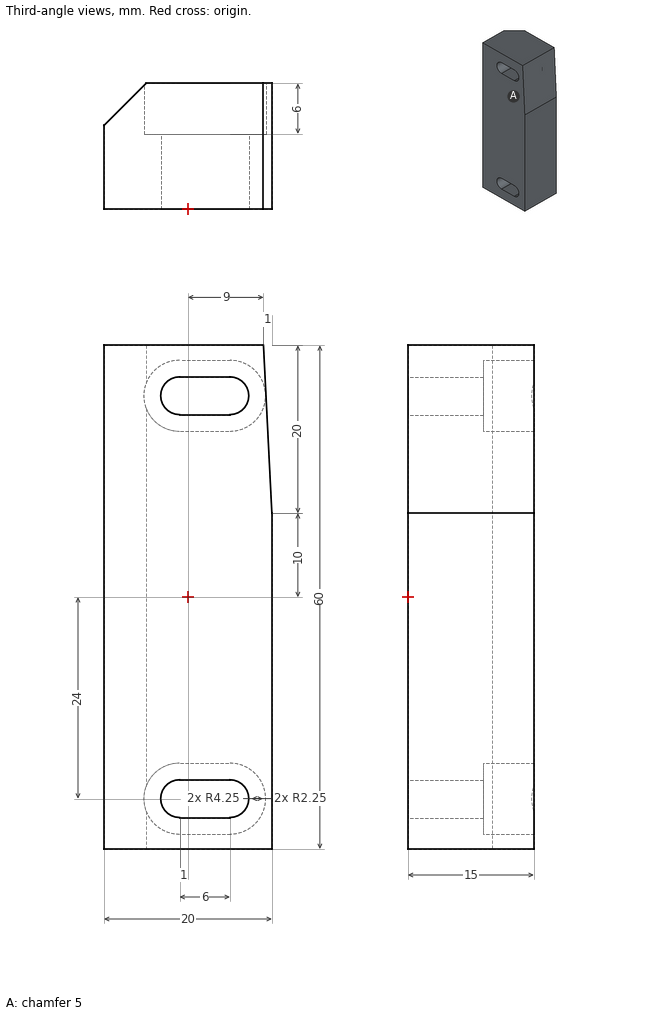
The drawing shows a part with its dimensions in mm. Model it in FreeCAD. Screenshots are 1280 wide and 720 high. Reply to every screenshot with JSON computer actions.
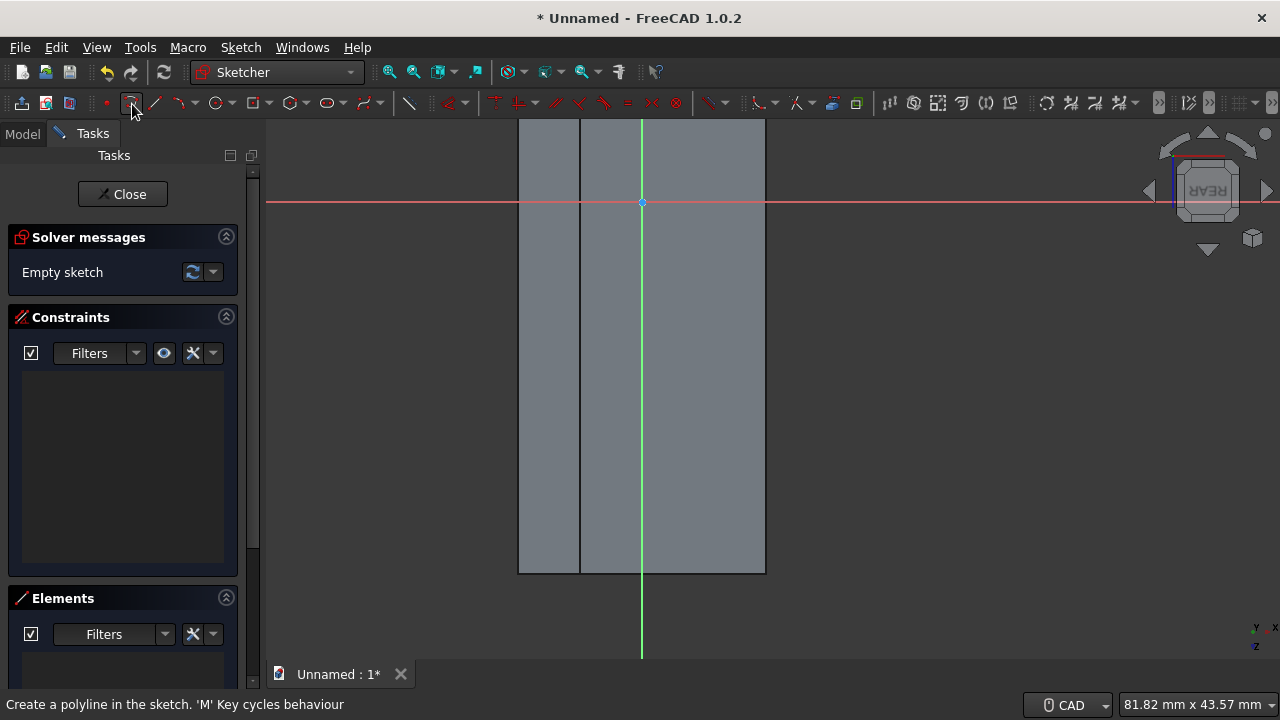
{"action": "left_click", "coordinate": [766, 326]}
{"action": "left_click", "coordinate": [753, 574]}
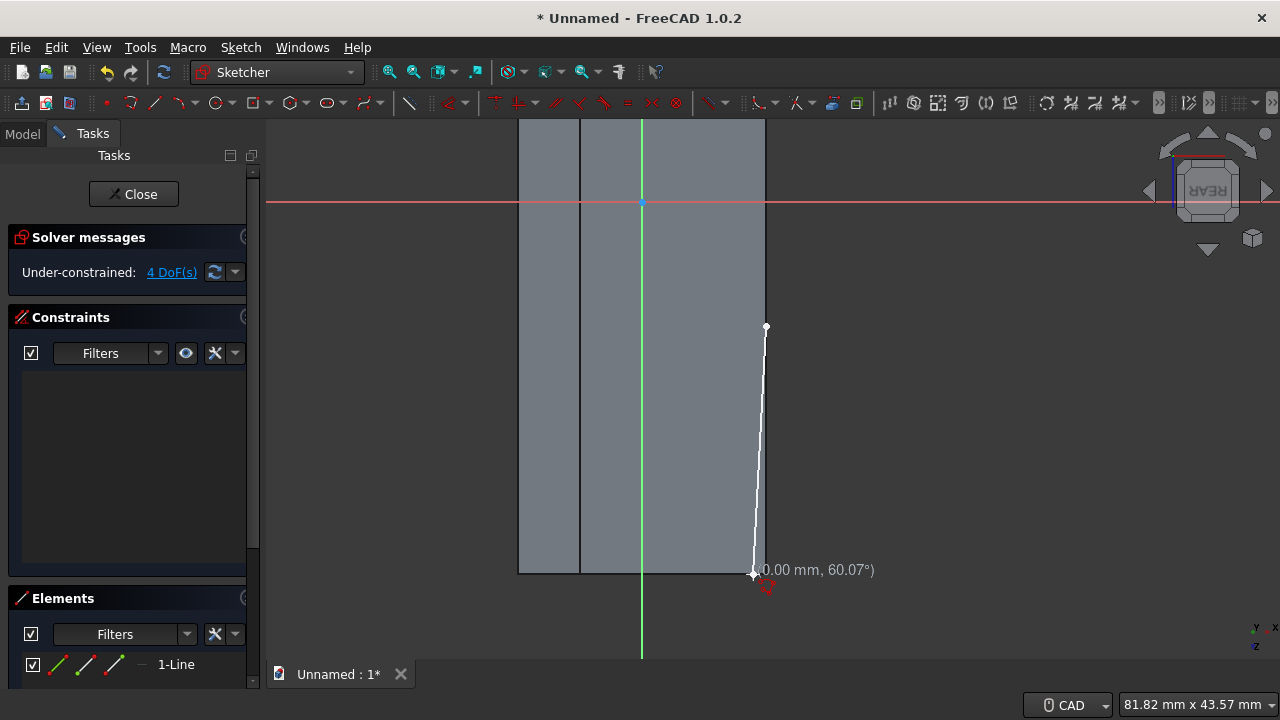
{"action": "scroll", "coordinate": [766, 574], "scroll_direction": "up", "scroll_amount": 2}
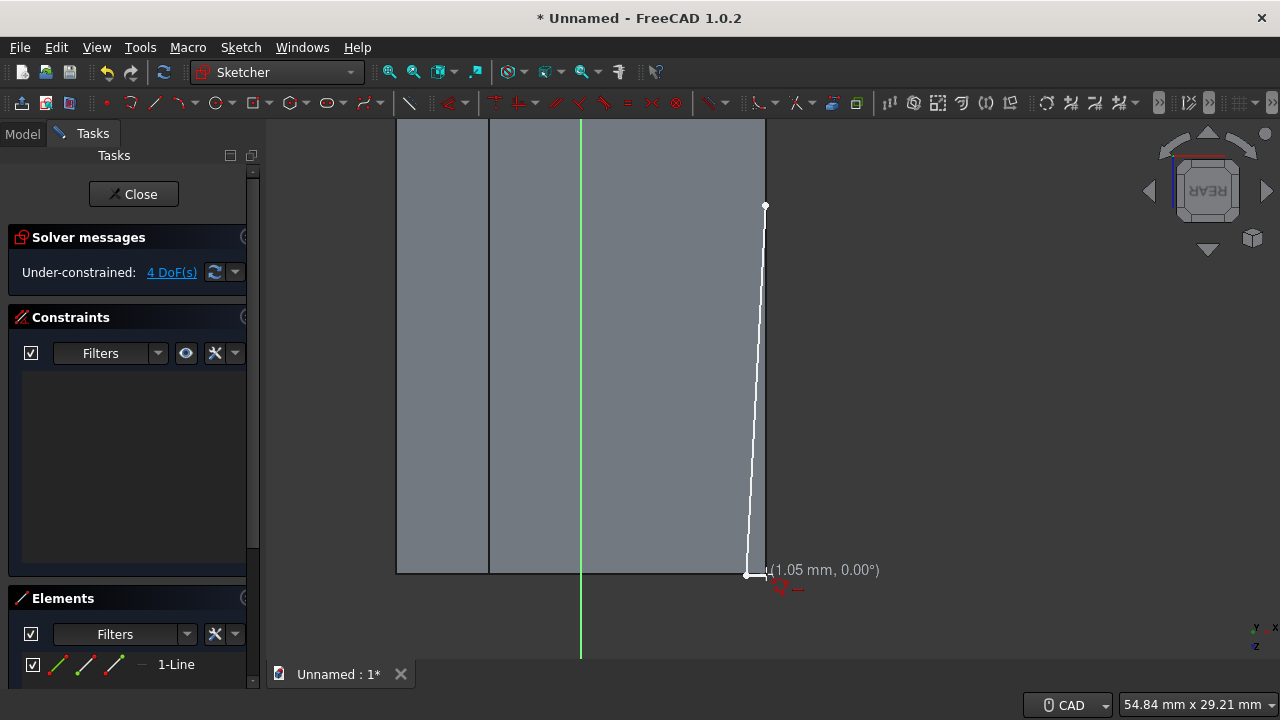
{"action": "left_click", "coordinate": [766, 574]}
{"action": "left_click", "coordinate": [766, 205]}
{"action": "key", "text": "Escape"}
{"action": "key", "text": "Escape"}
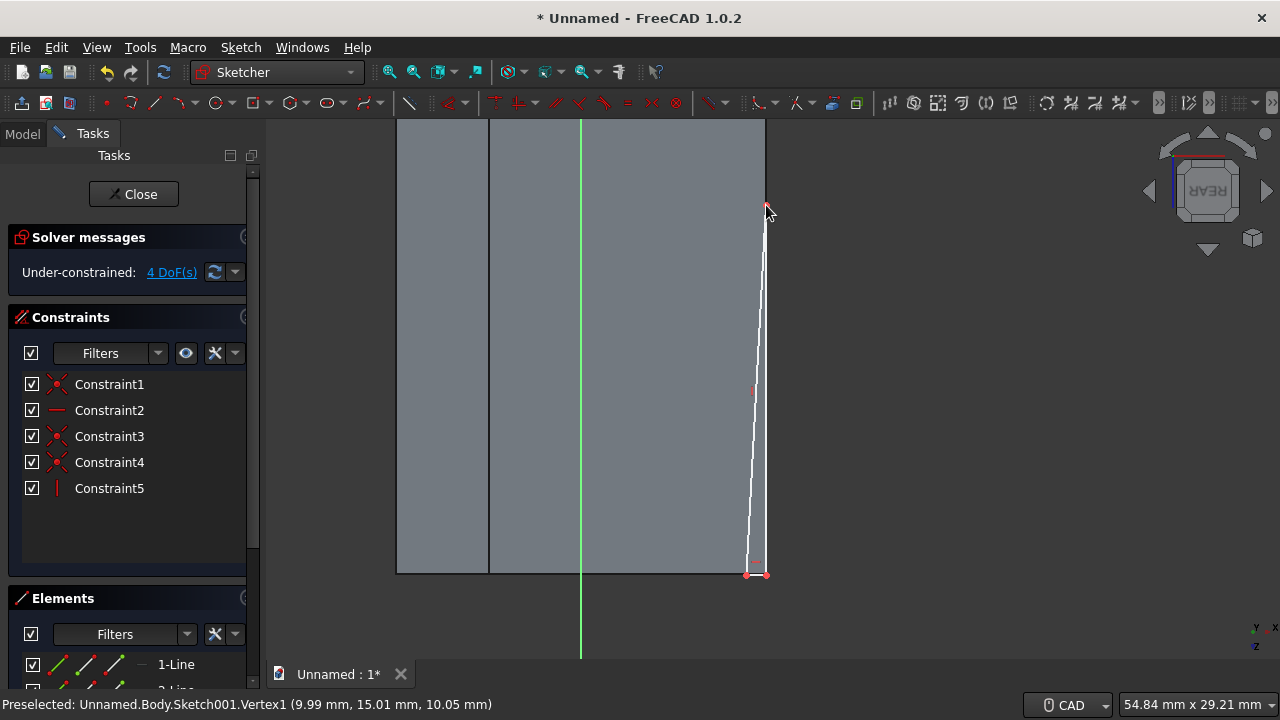
{"action": "left_click", "coordinate": [448, 104]}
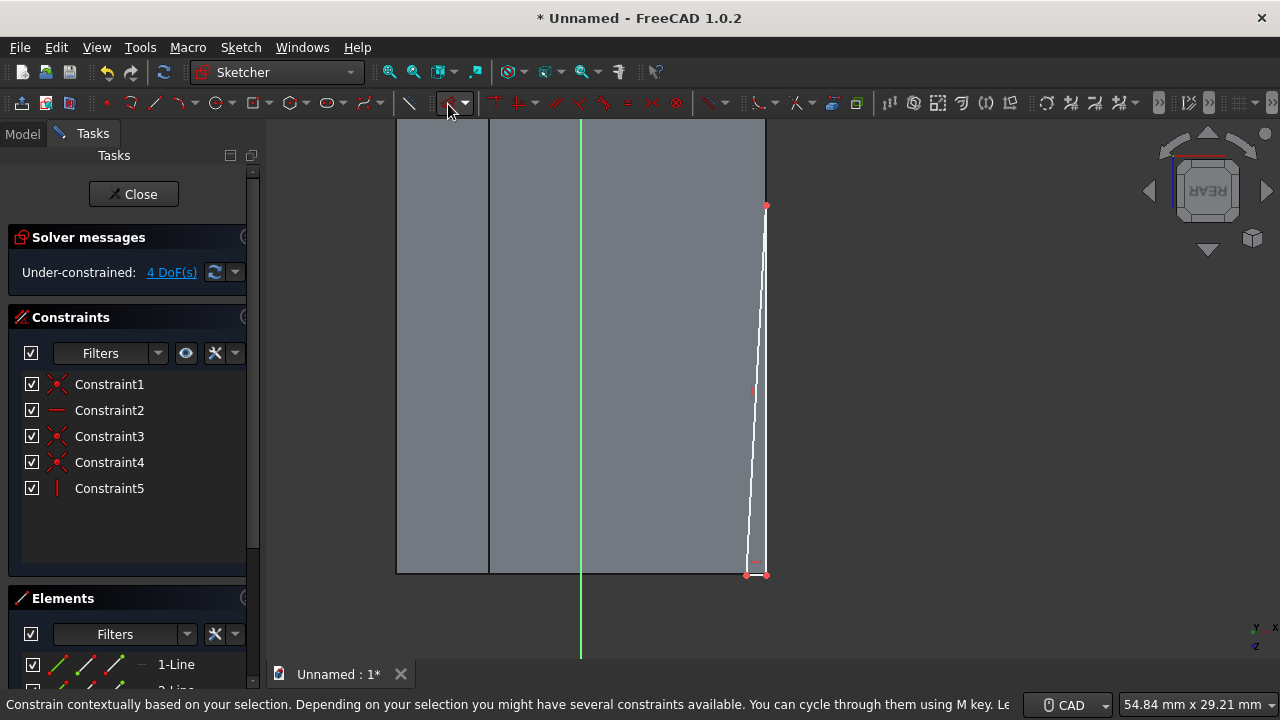
{"action": "scroll", "coordinate": [756, 575], "scroll_direction": "up", "scroll_amount": 4}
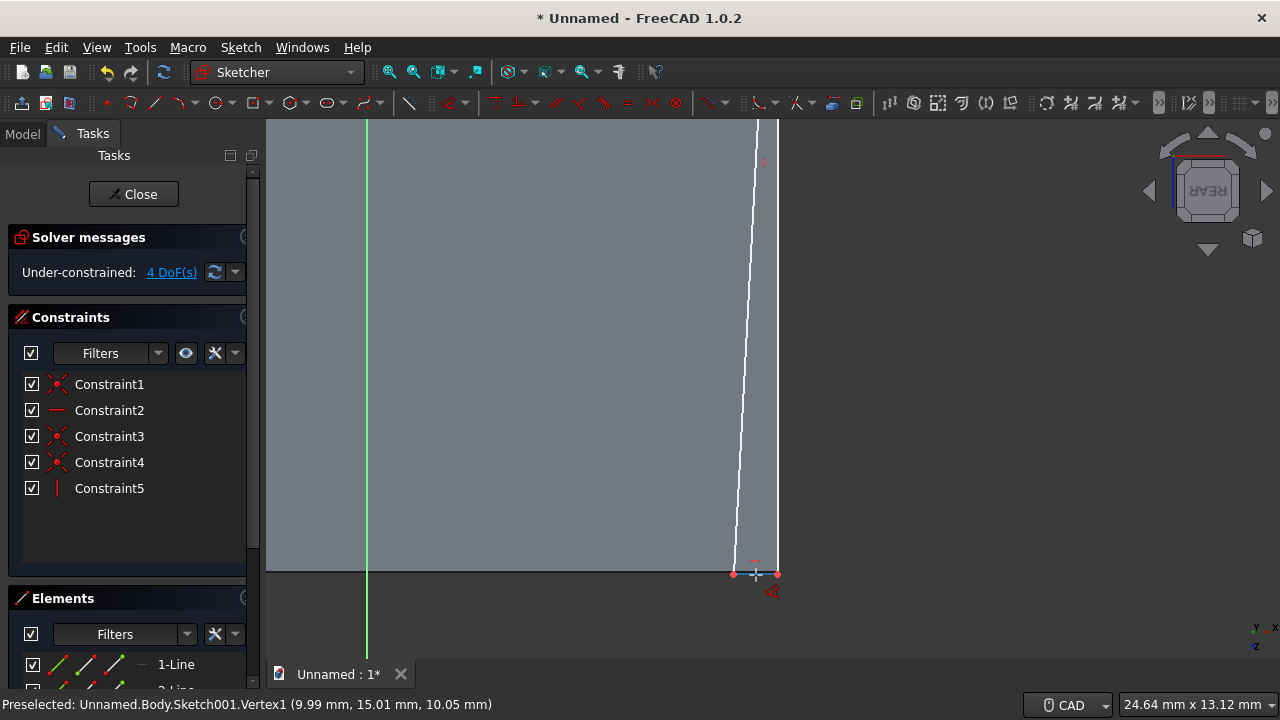
{"action": "left_click", "coordinate": [756, 574]}
{"action": "left_click", "coordinate": [756, 608]}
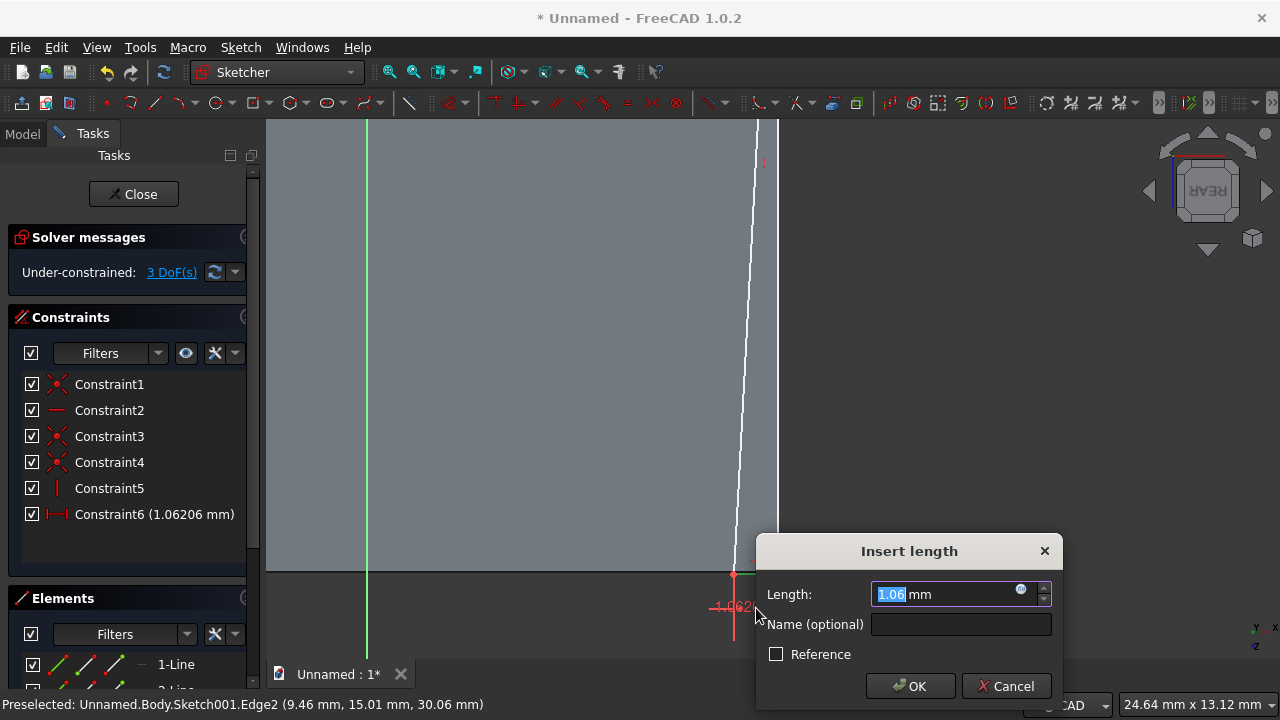
{"action": "type", "text": "1"}
{"action": "key", "text": "Return"}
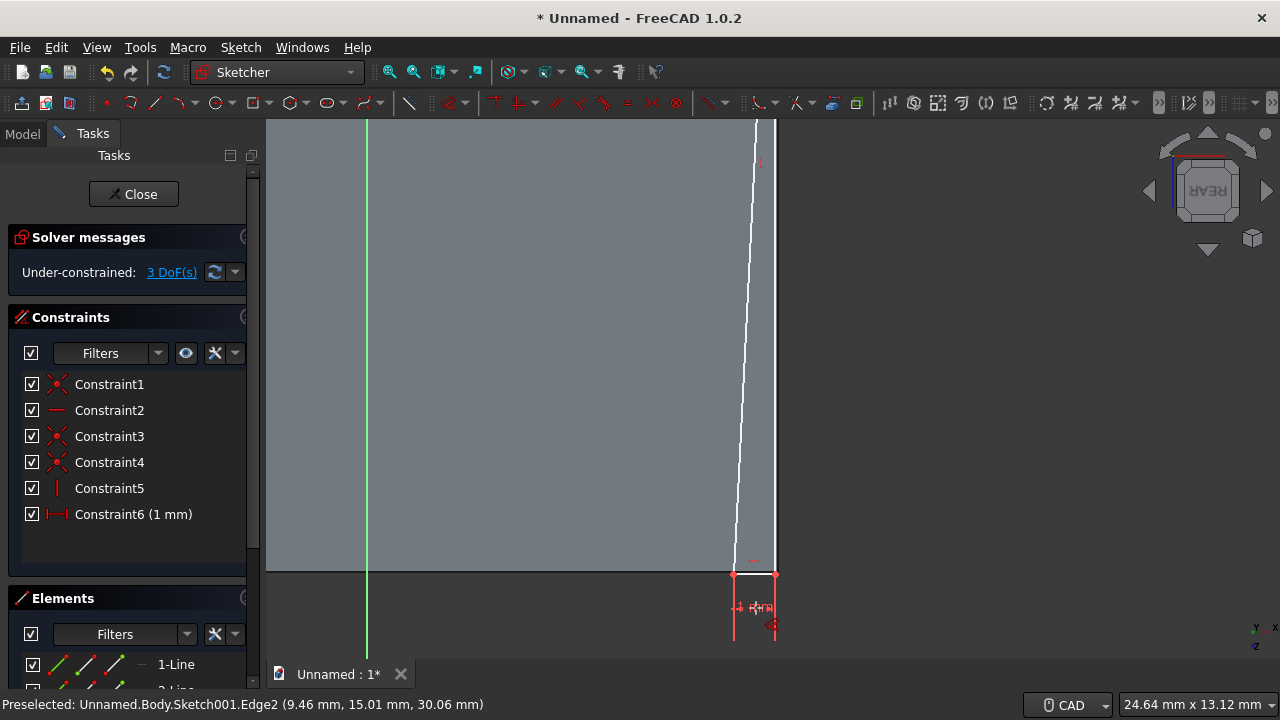
{"action": "left_click", "coordinate": [775, 327]}
{"action": "left_click", "coordinate": [809, 361]}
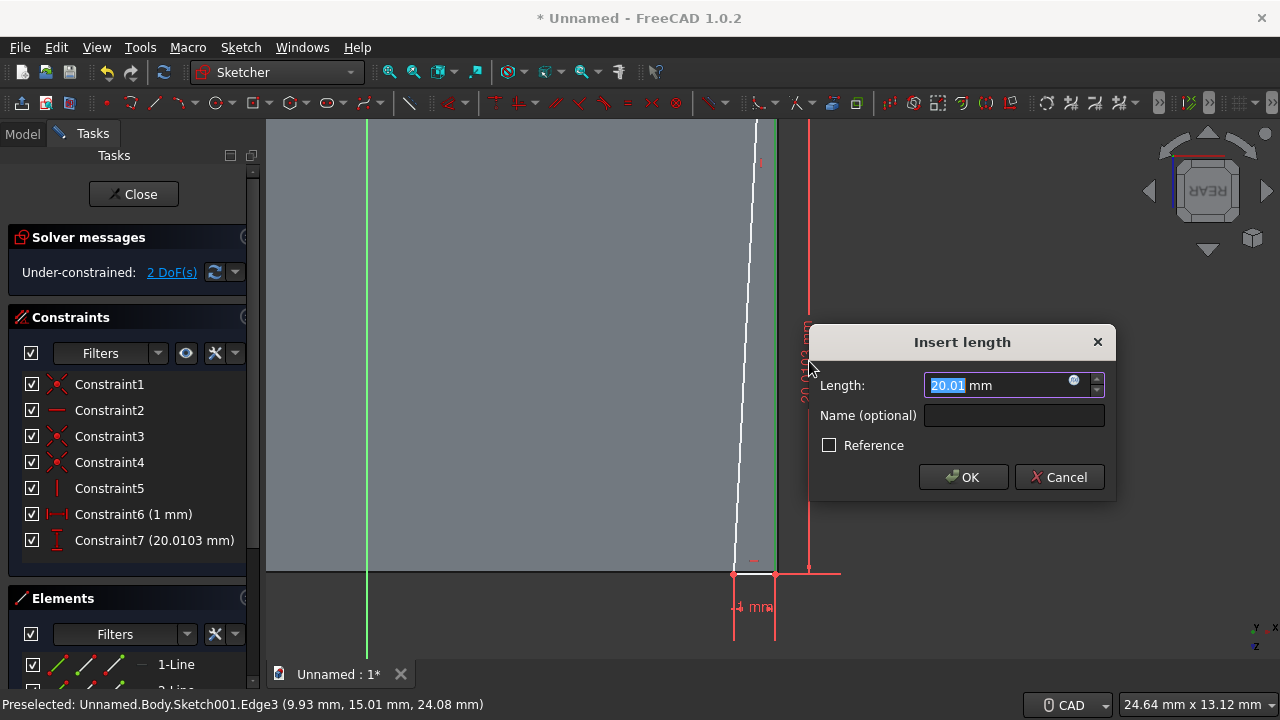
{"action": "type", "text": "20"}
{"action": "key", "text": "Return"}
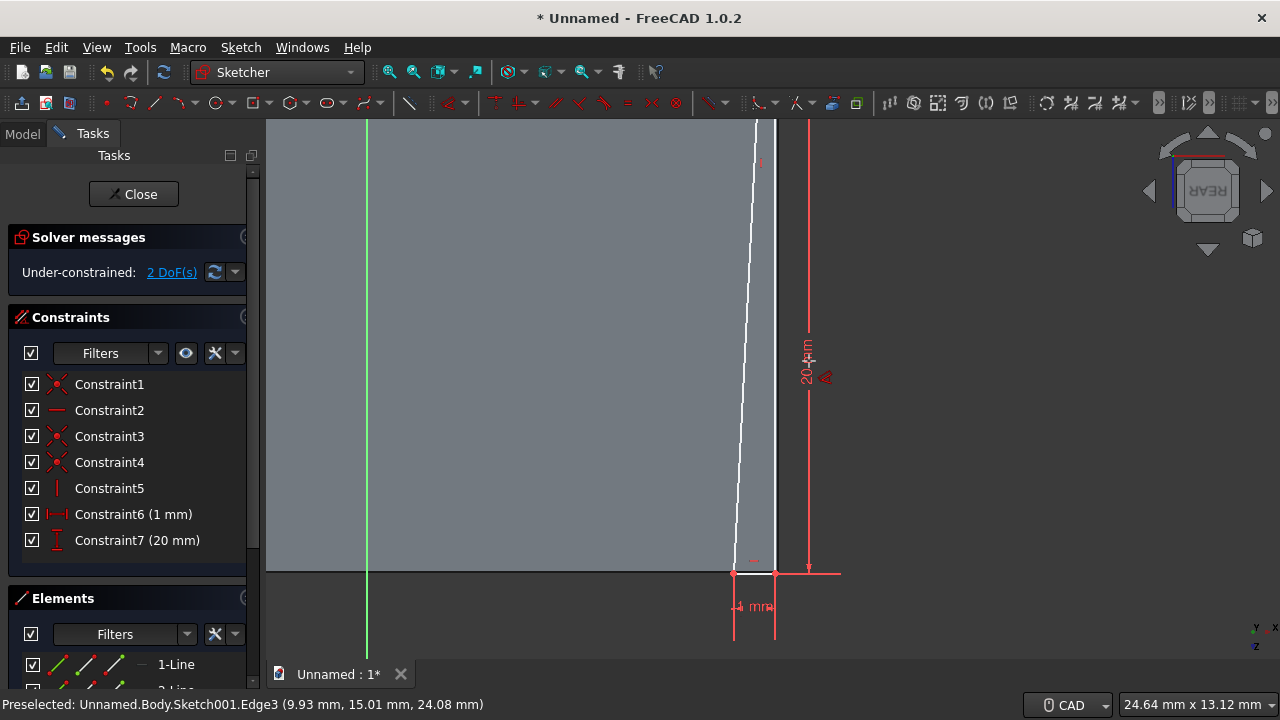
{"action": "left_click", "coordinate": [734, 574]}
{"action": "left_click", "coordinate": [550, 608]}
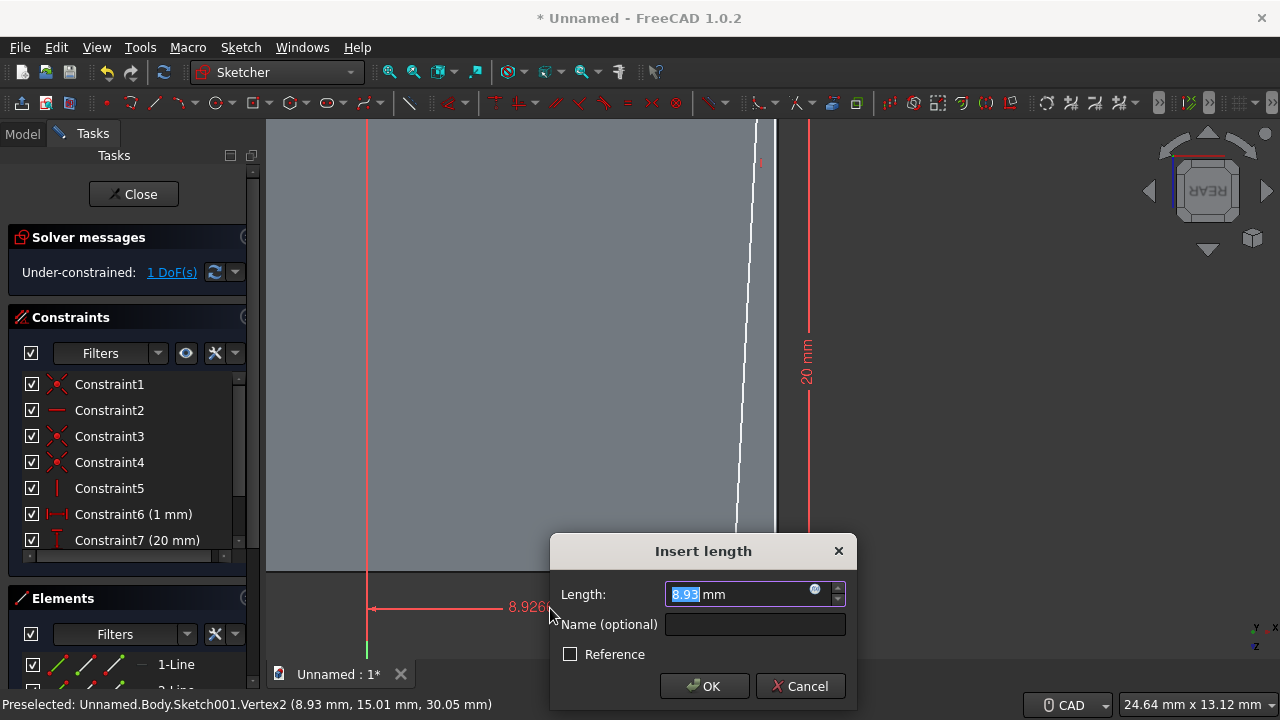
{"action": "type", "text": "9"}
{"action": "key", "text": "Return"}